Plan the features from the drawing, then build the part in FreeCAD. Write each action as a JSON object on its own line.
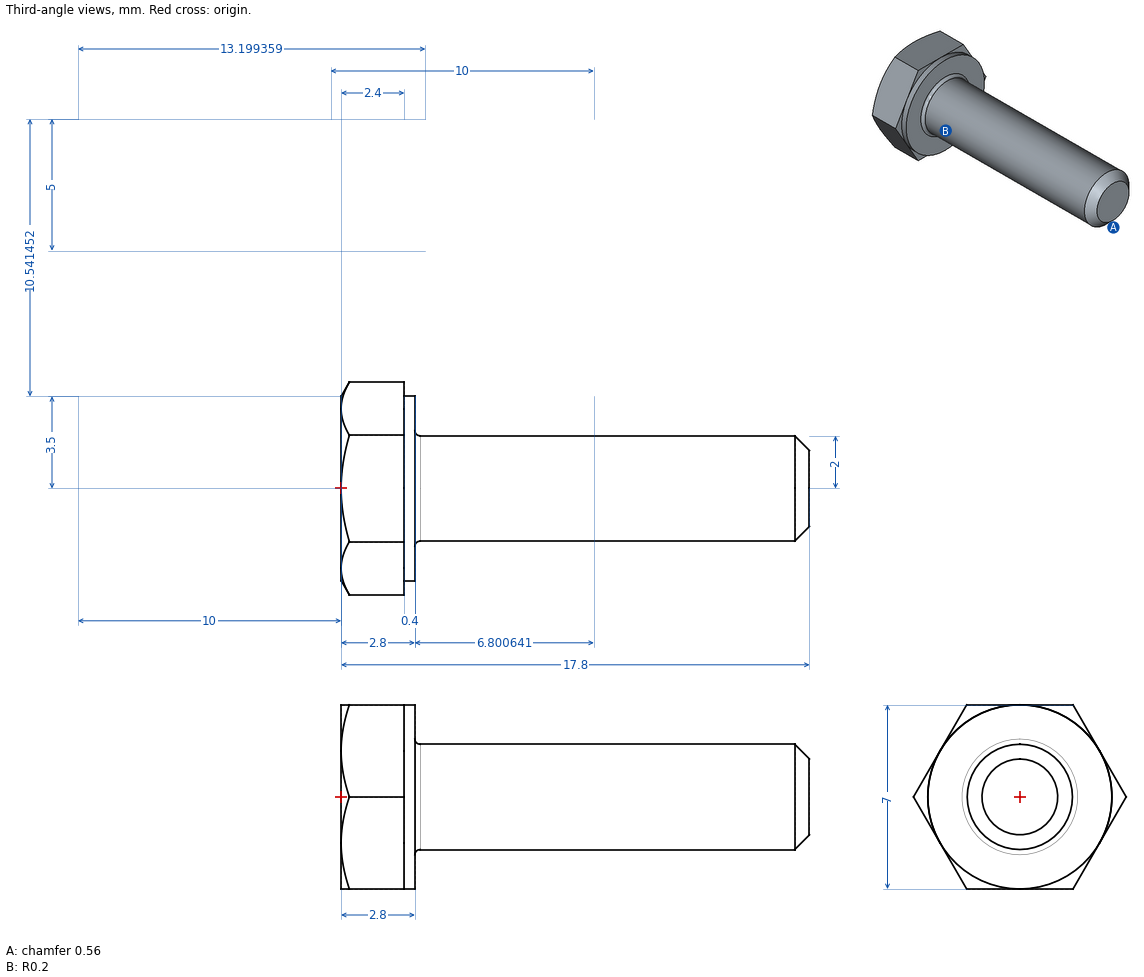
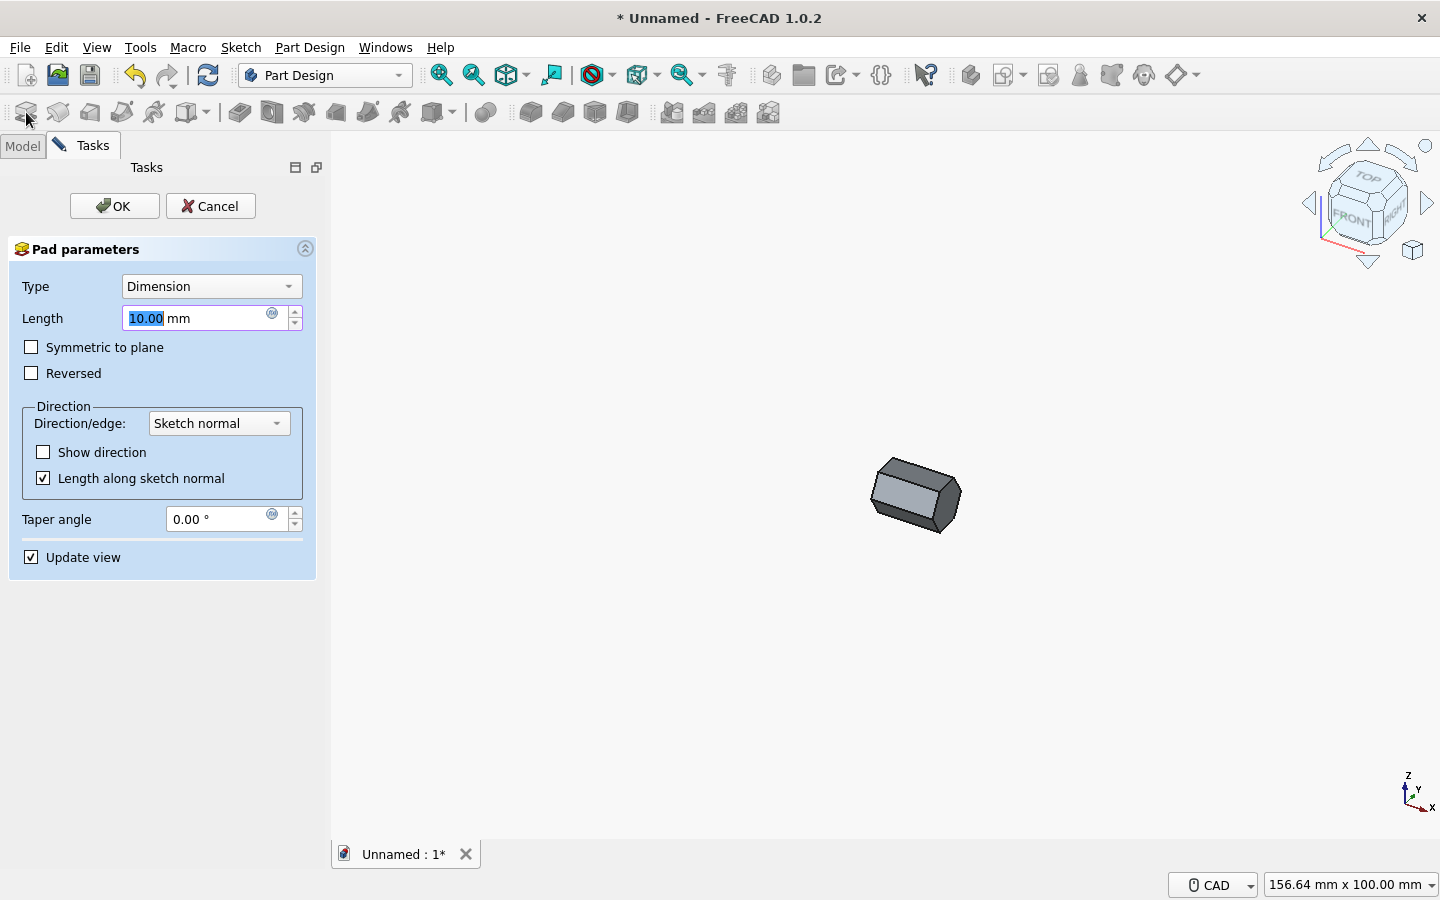
{"action": "type", "text": "2.8"}
{"action": "key", "text": "Tab"}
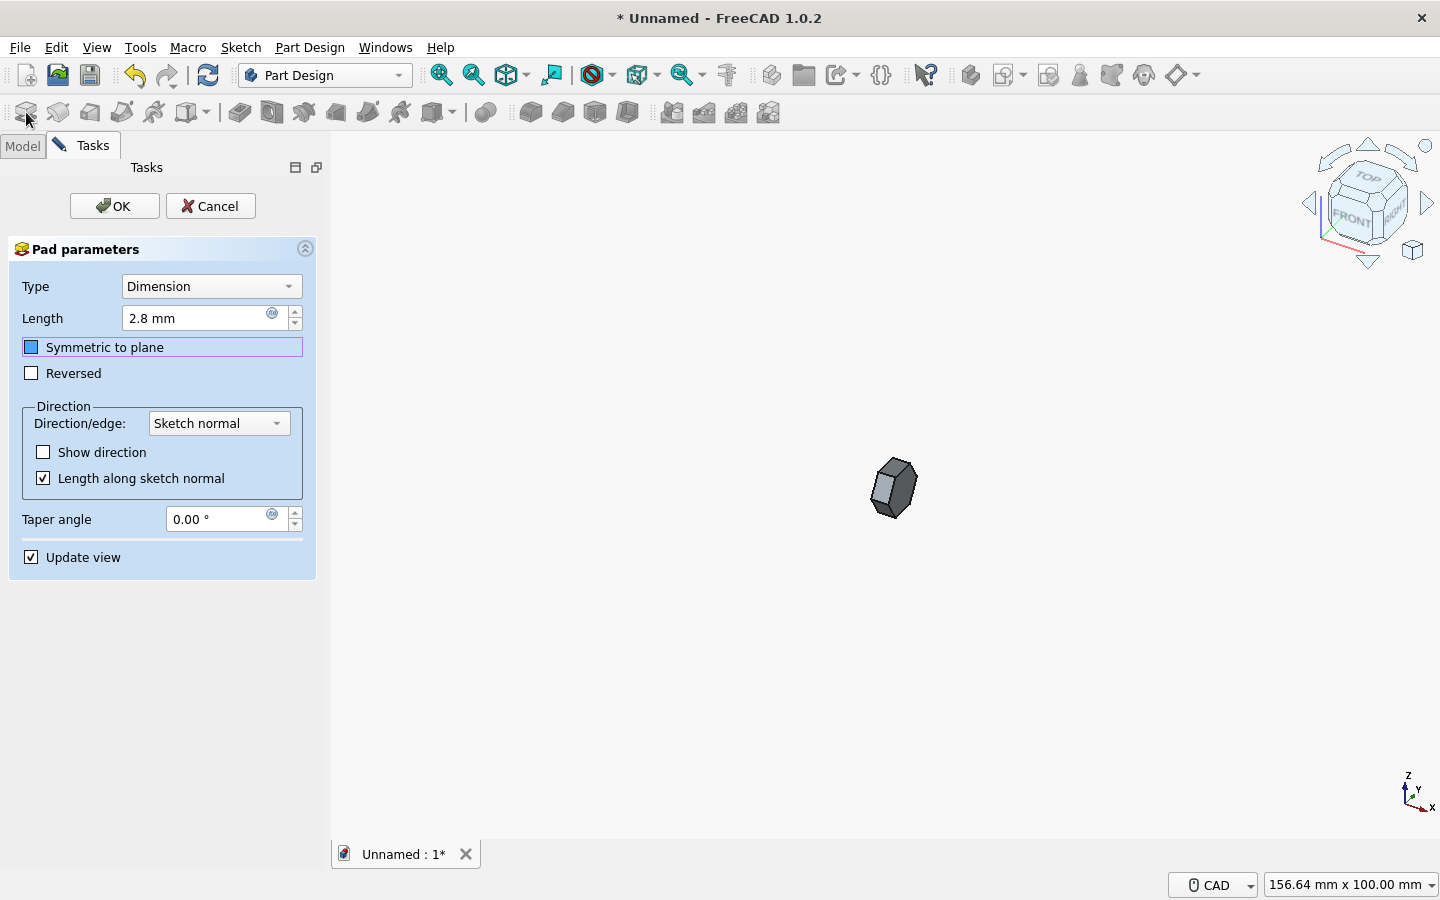
{"action": "left_click", "coordinate": [115, 206]}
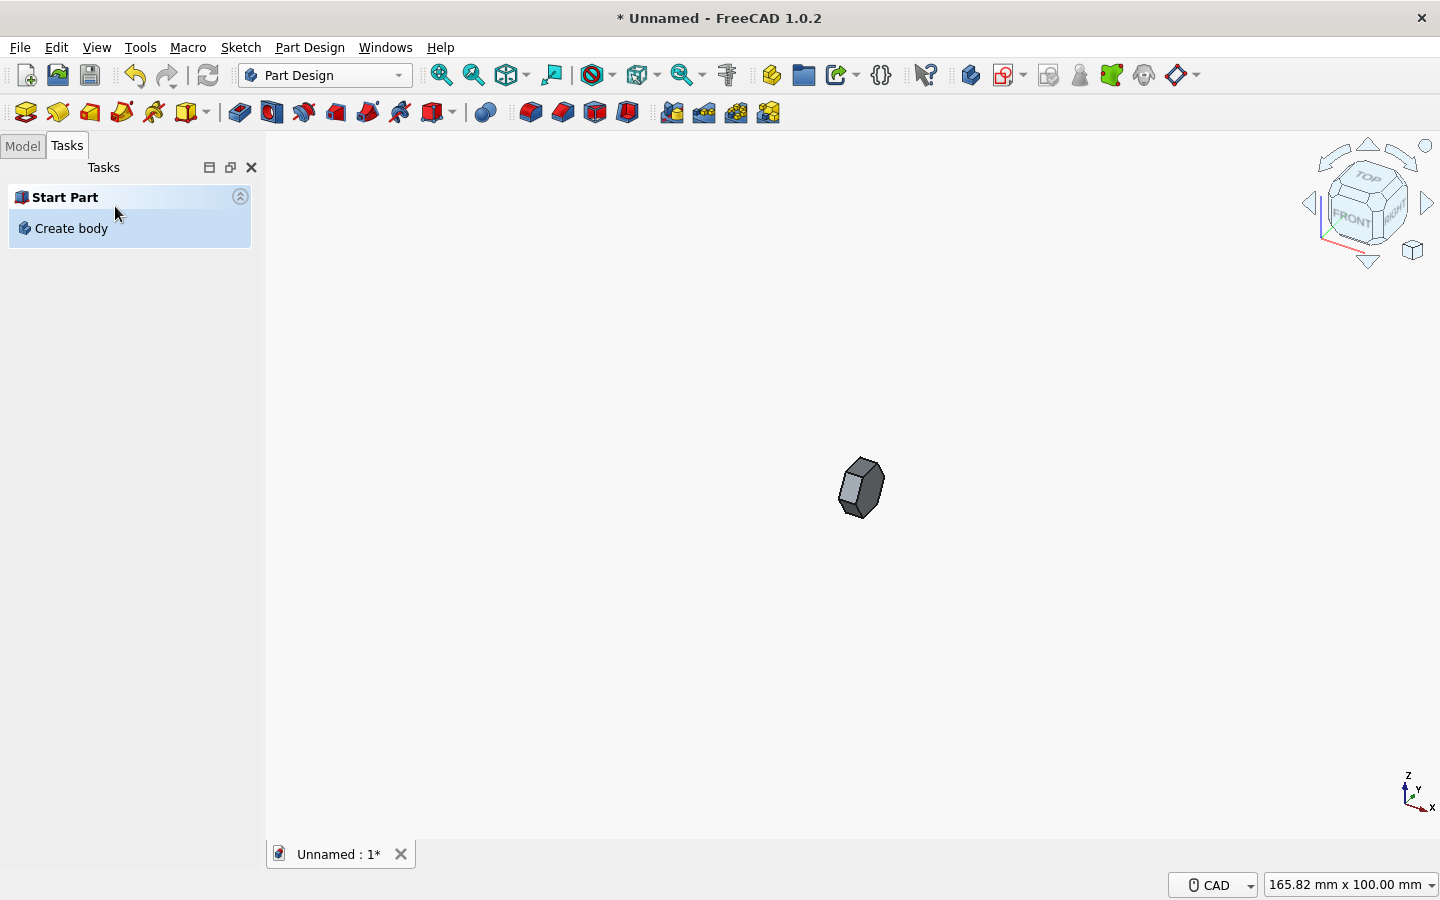
{"action": "key", "text": "v f"}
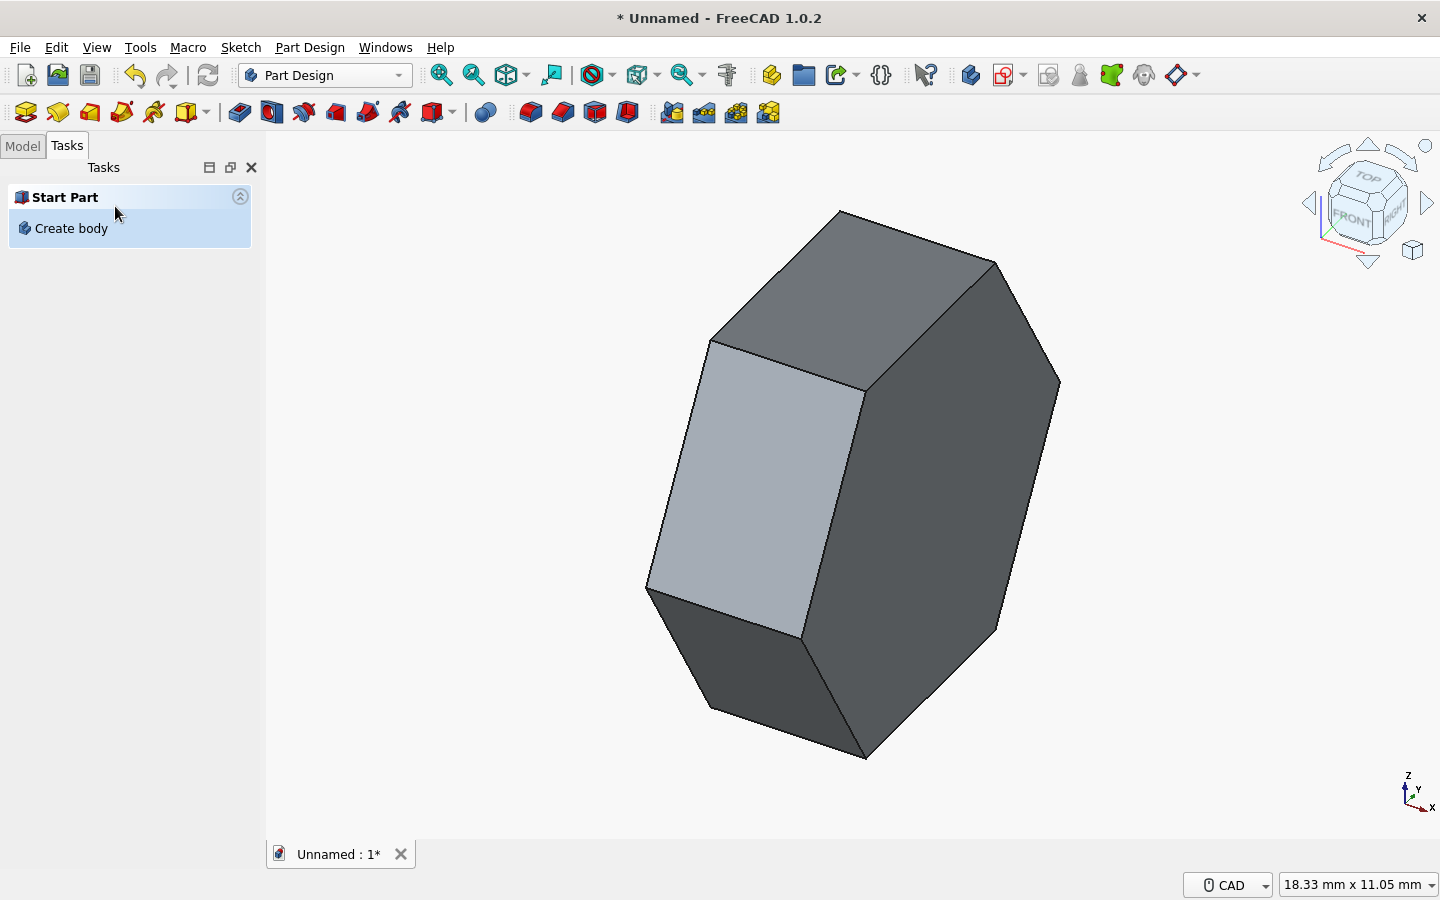
{"action": "left_click", "coordinate": [1004, 76]}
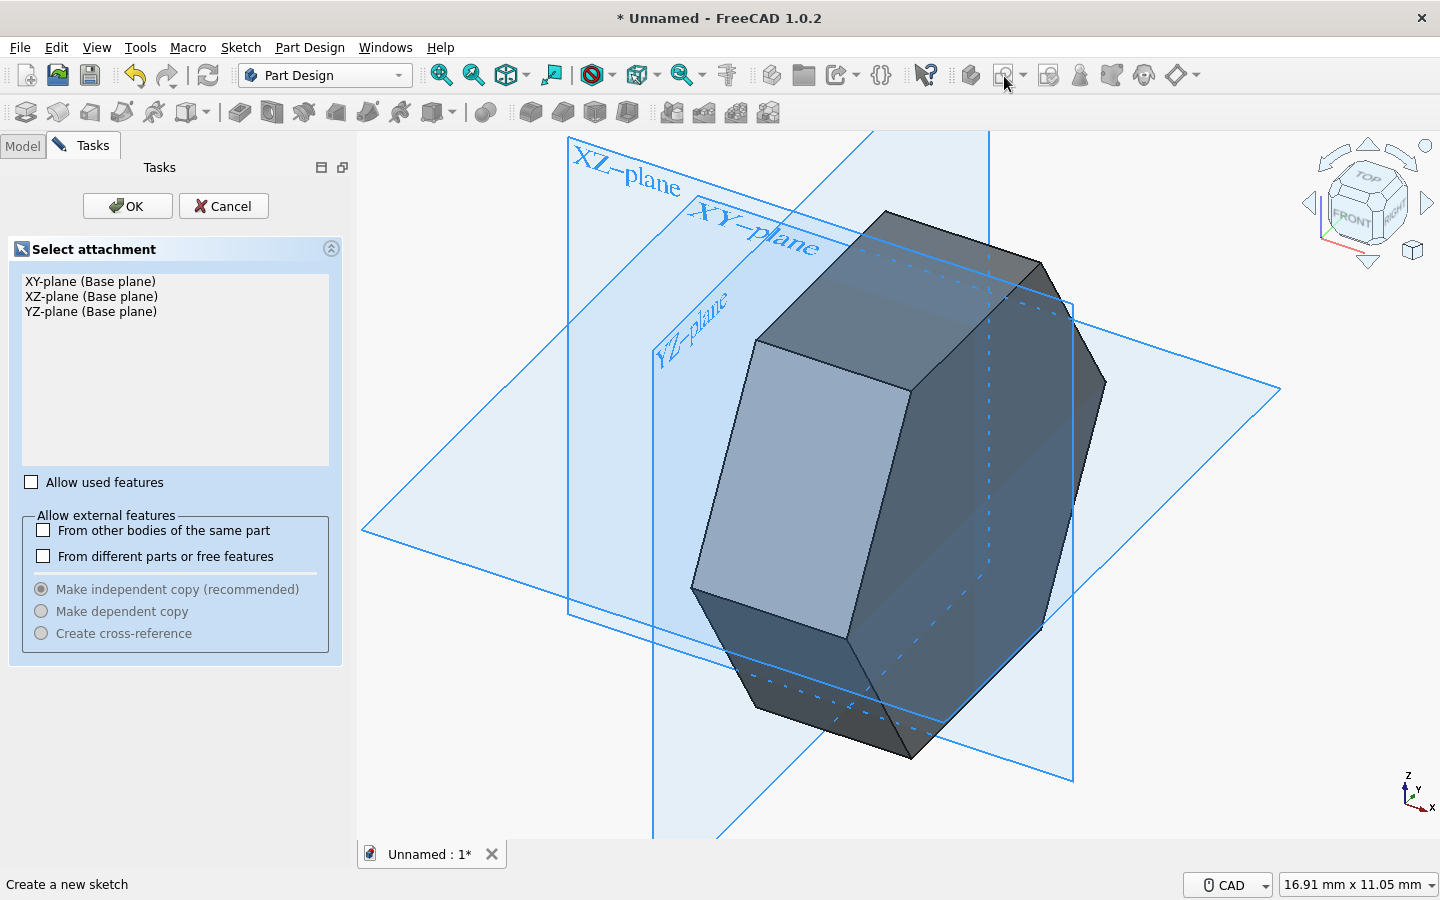
{"action": "left_click", "coordinate": [82, 282]}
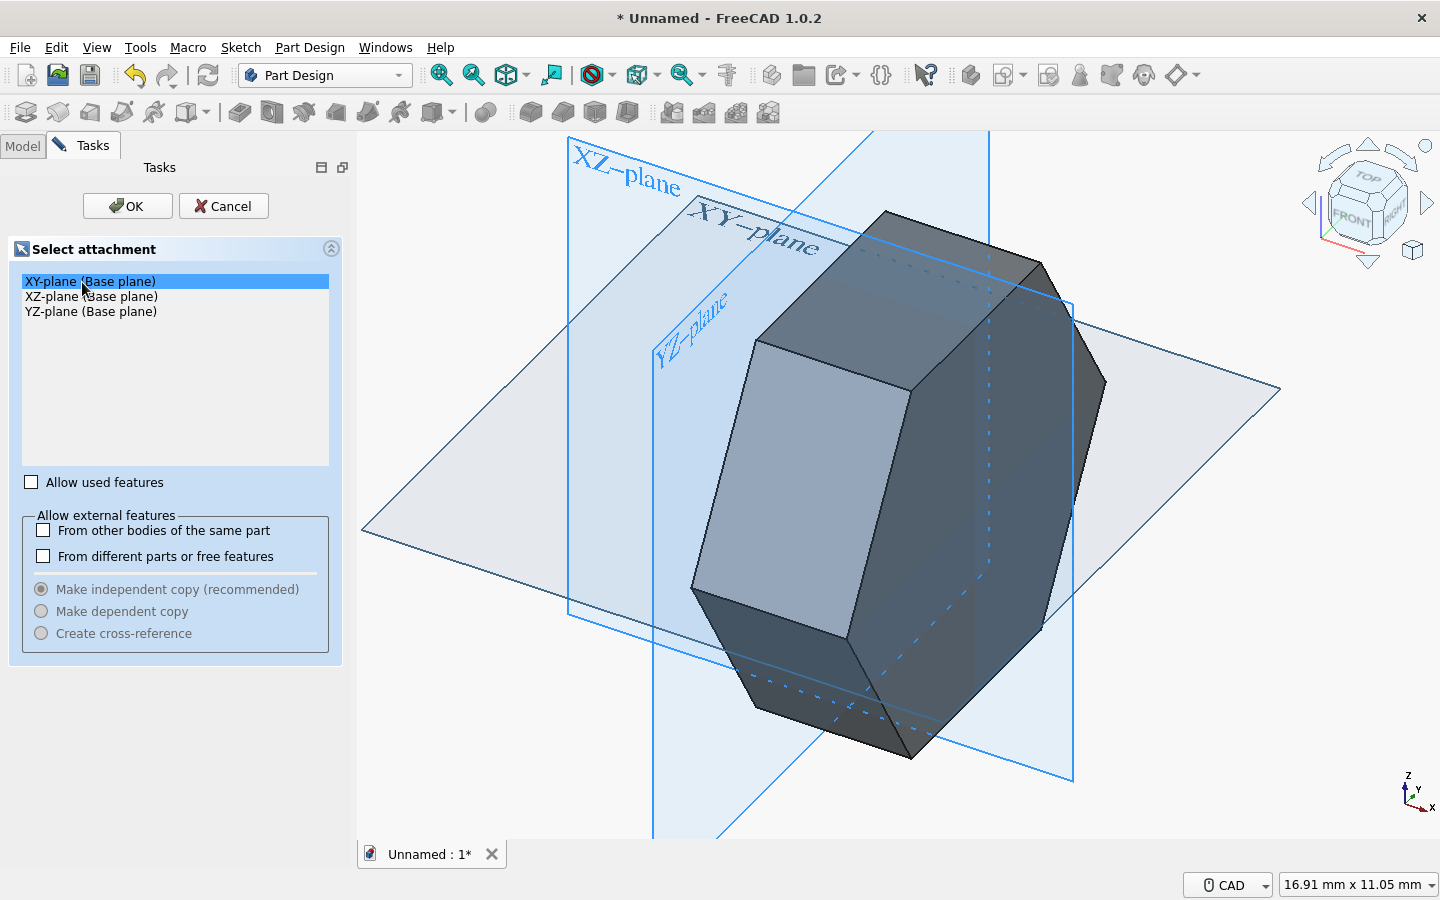
{"action": "left_click", "coordinate": [128, 206]}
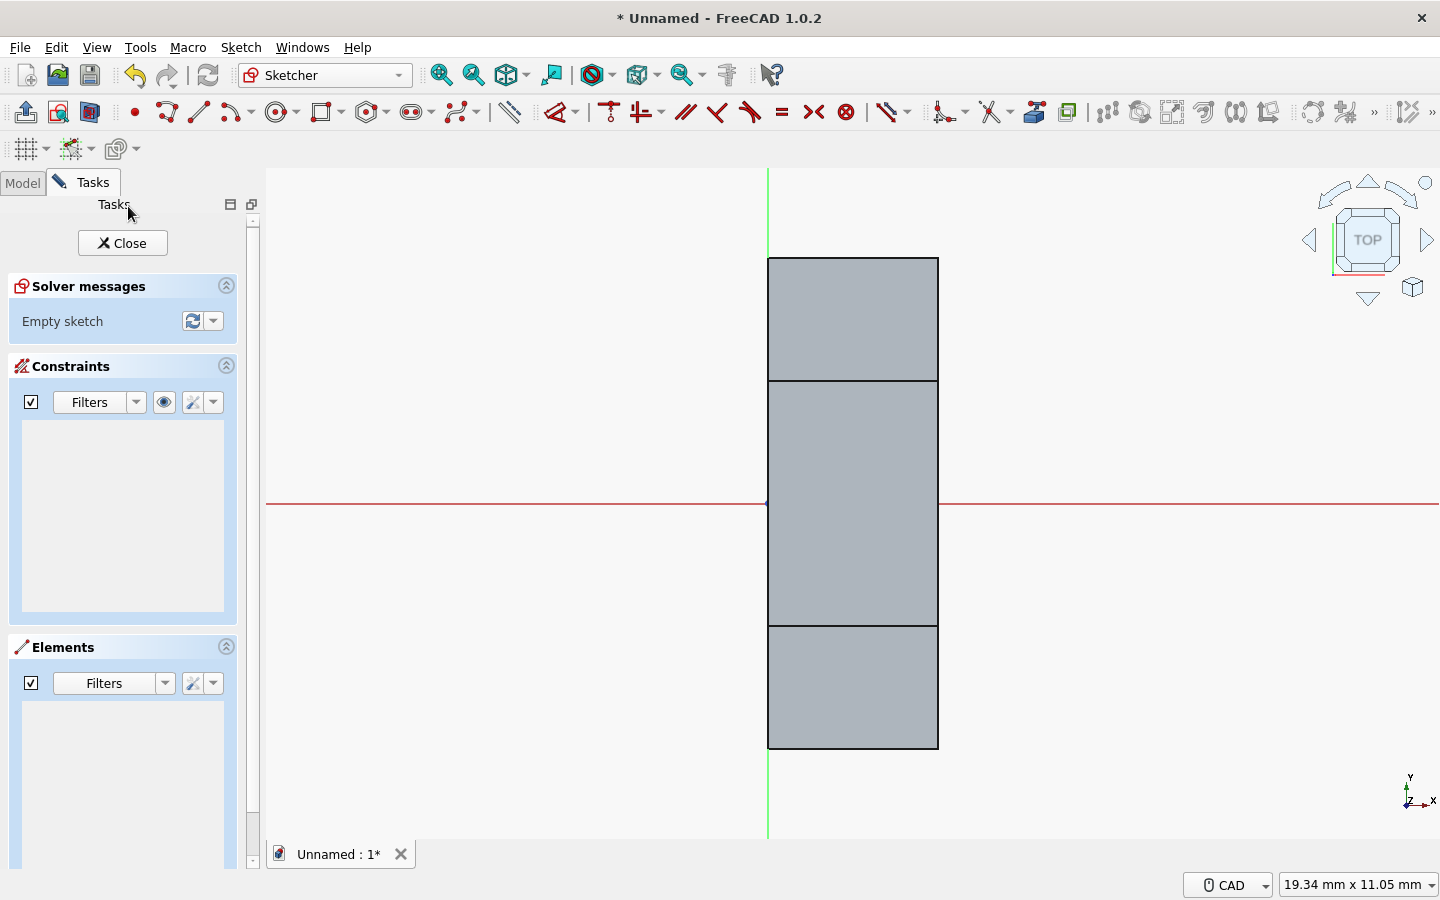
{"action": "key", "text": "q s"}